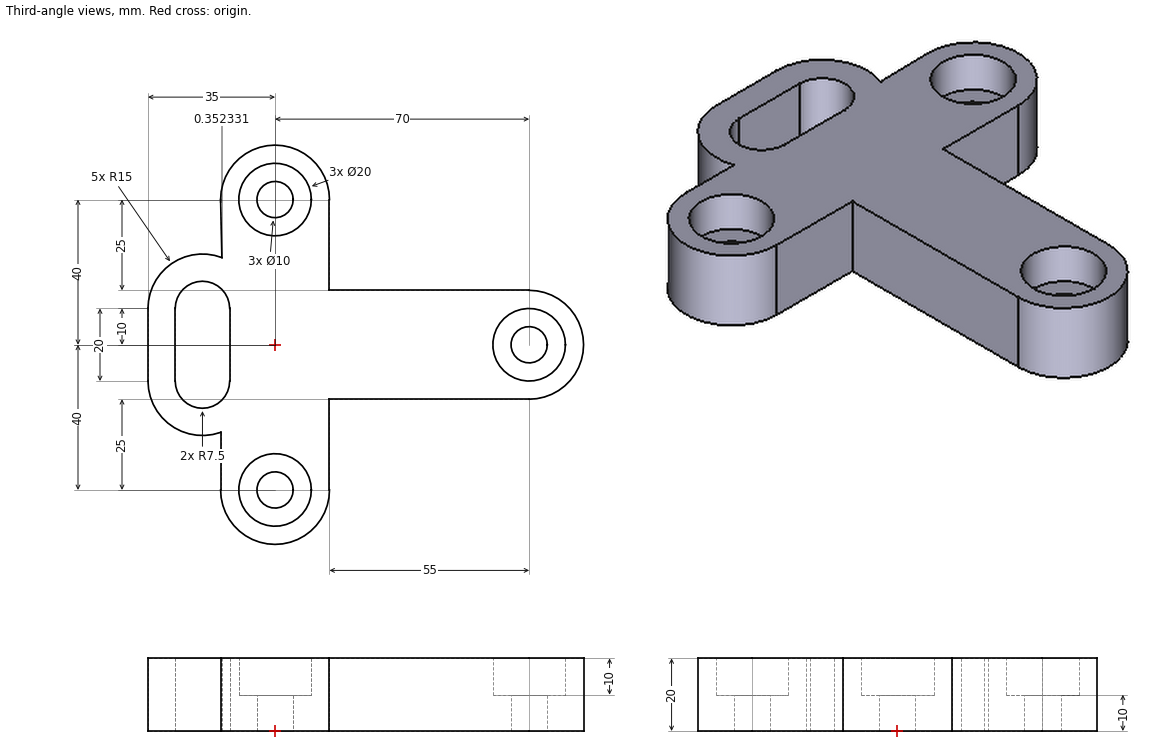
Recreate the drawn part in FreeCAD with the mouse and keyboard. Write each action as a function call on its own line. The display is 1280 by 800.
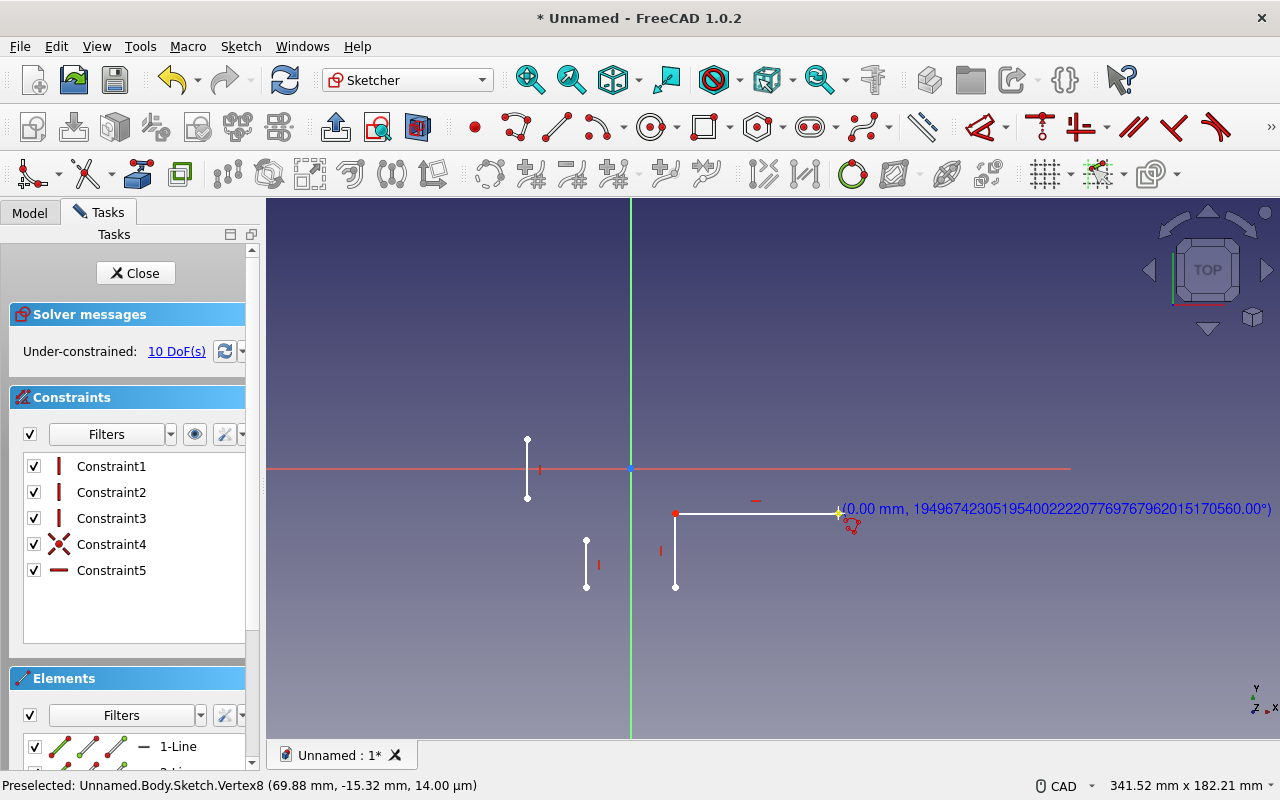
click(838, 424)
click(675, 424)
click(675, 350)
right_click(675, 350)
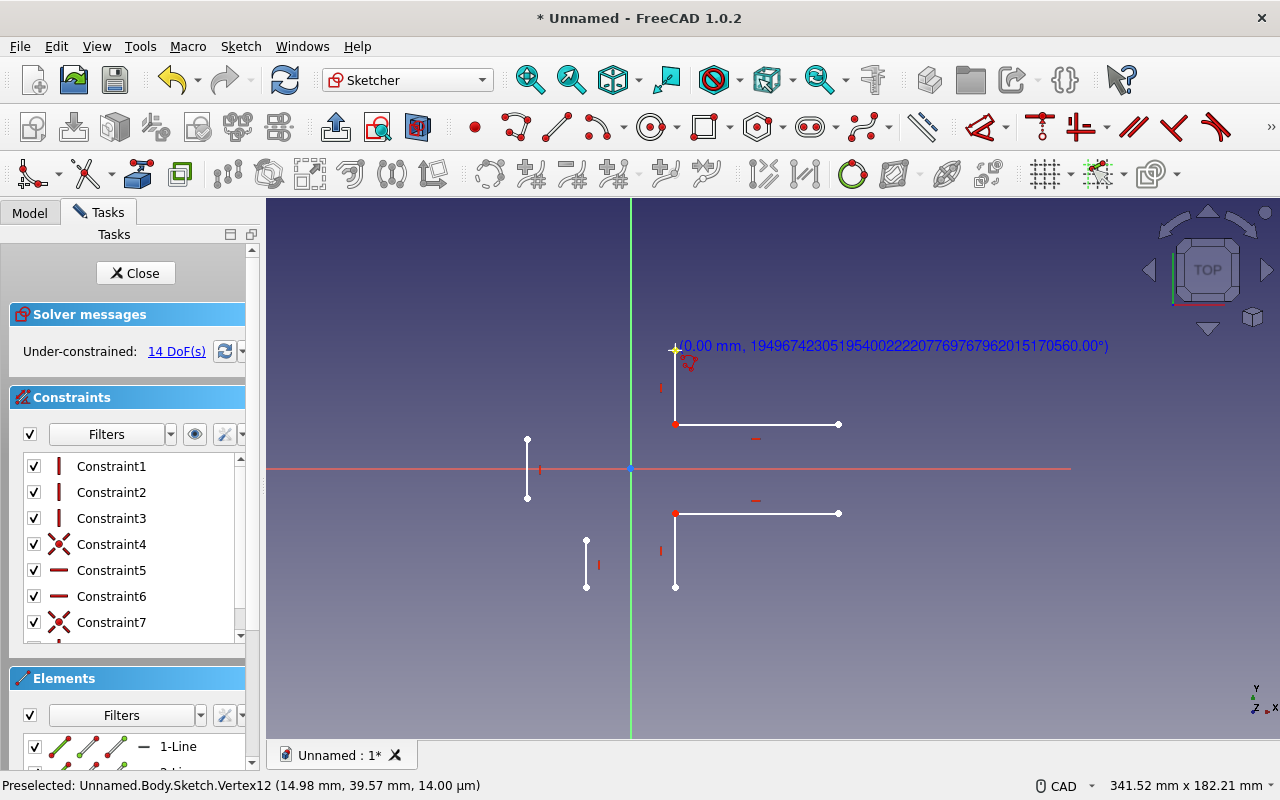
click(557, 128)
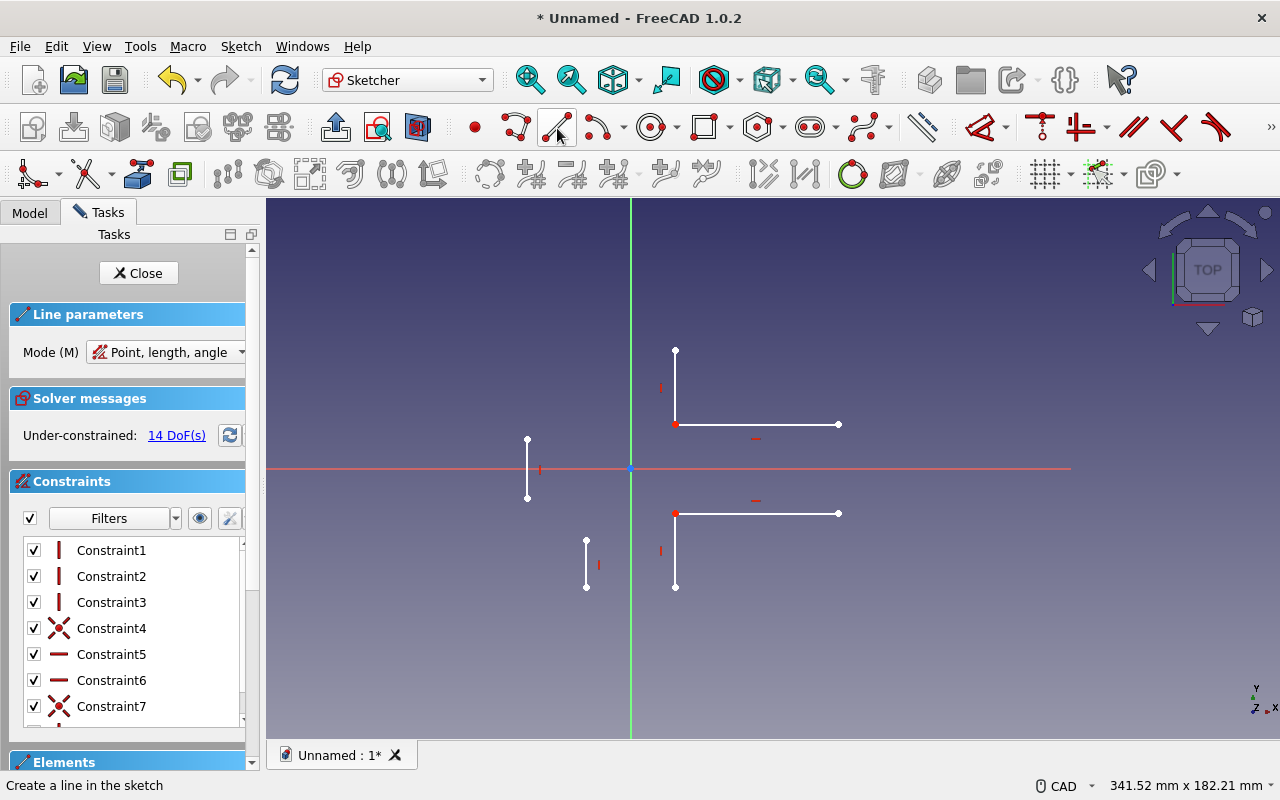
click(586, 350)
click(590, 397)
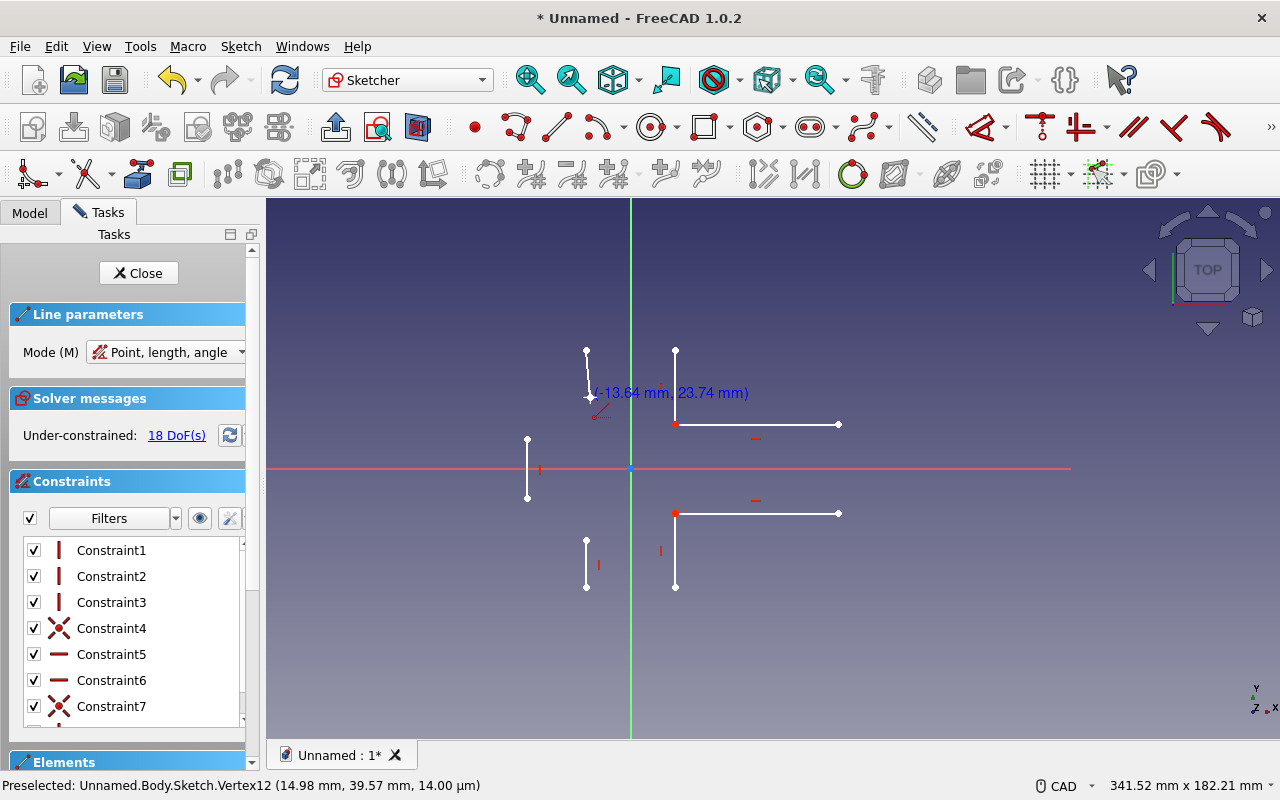
click(624, 128)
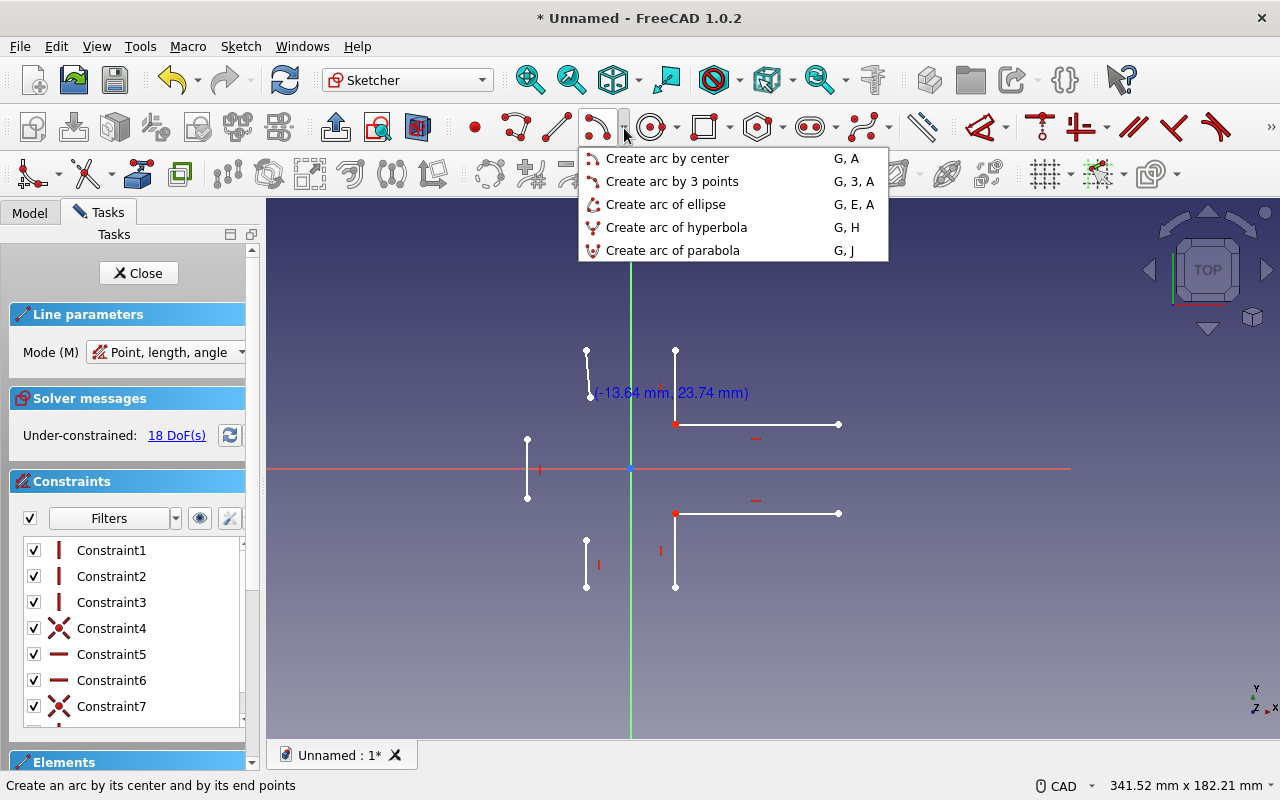
click(734, 182)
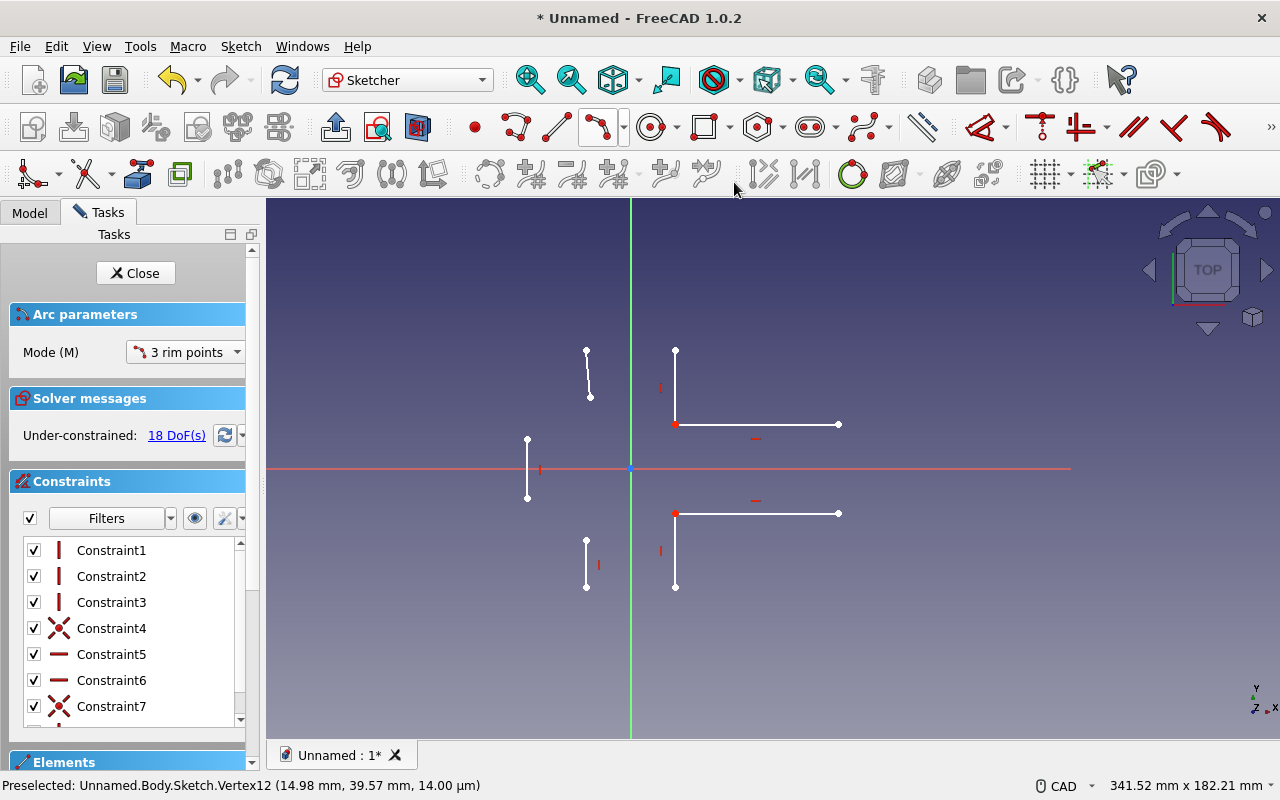
click(527, 499)
click(586, 541)
click(545, 535)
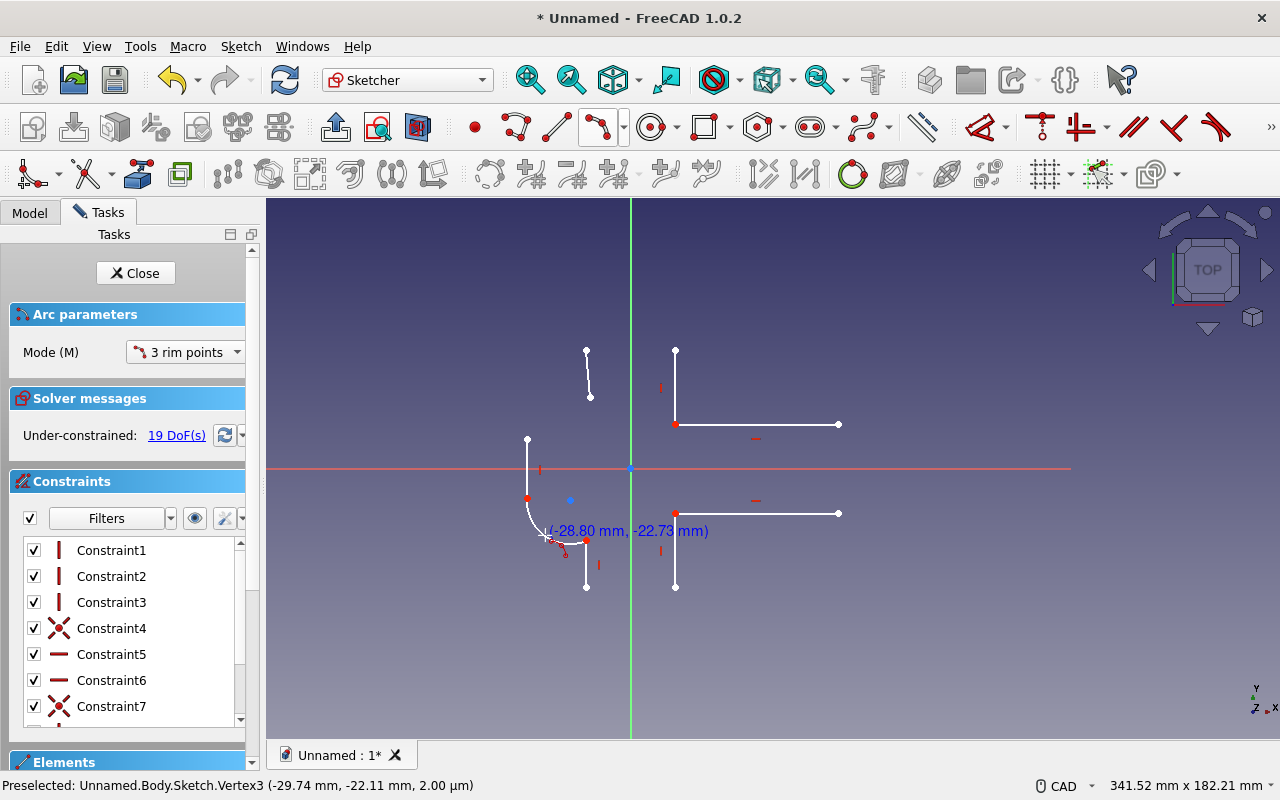
click(586, 588)
click(675, 588)
click(604, 623)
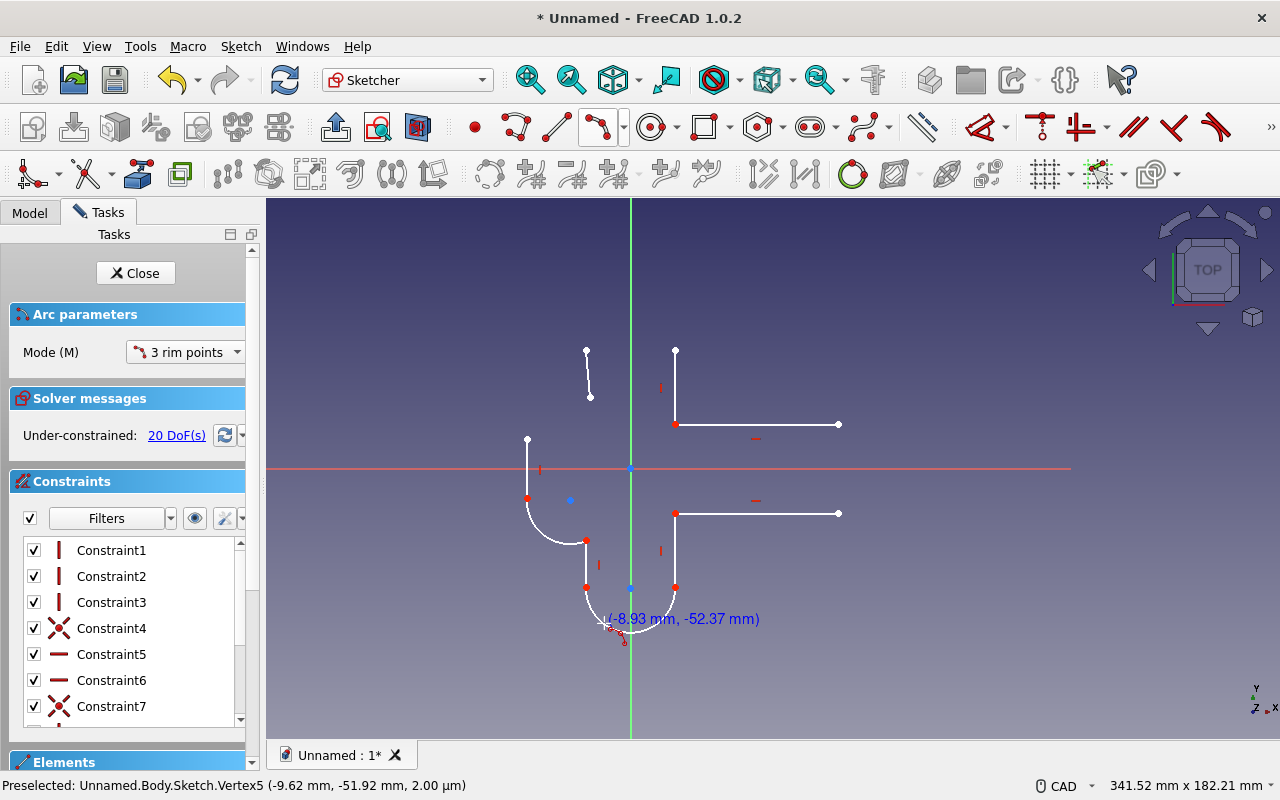
click(838, 514)
click(838, 425)
click(874, 495)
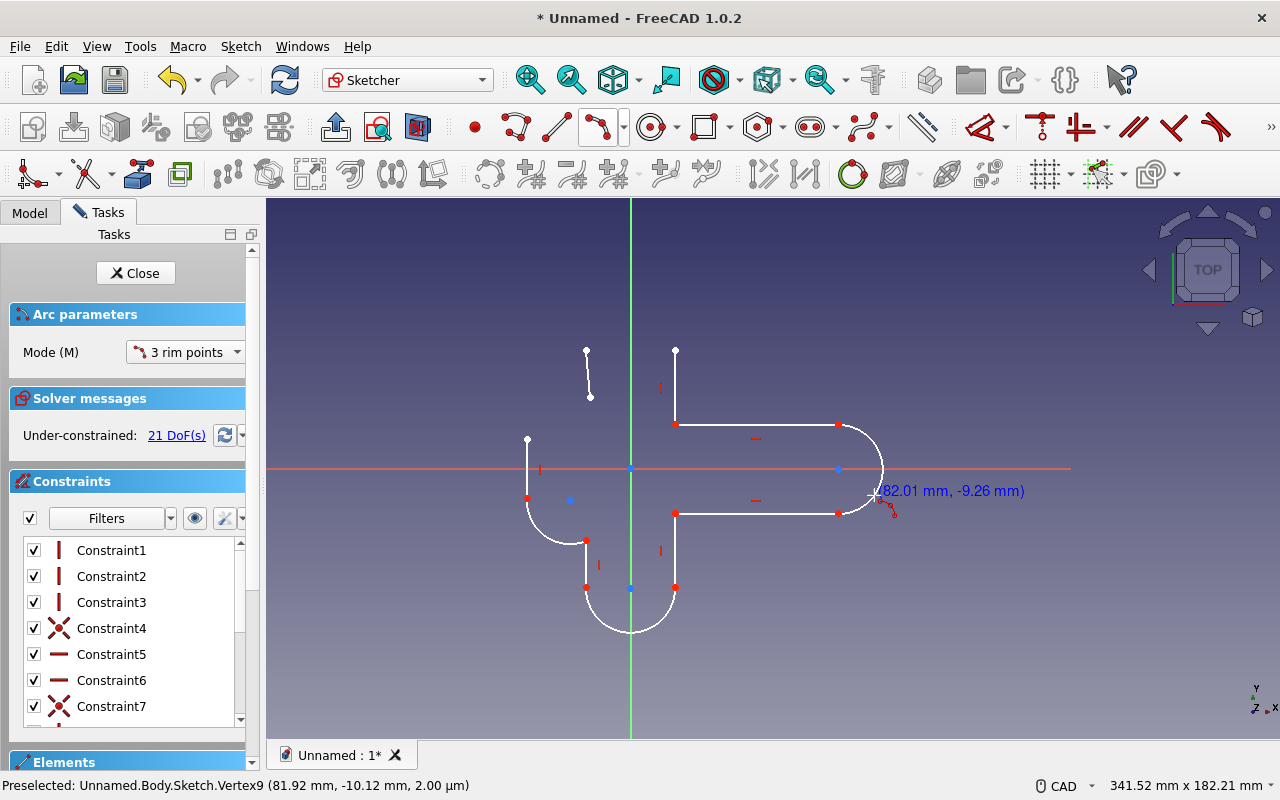
click(675, 351)
click(586, 351)
click(657, 314)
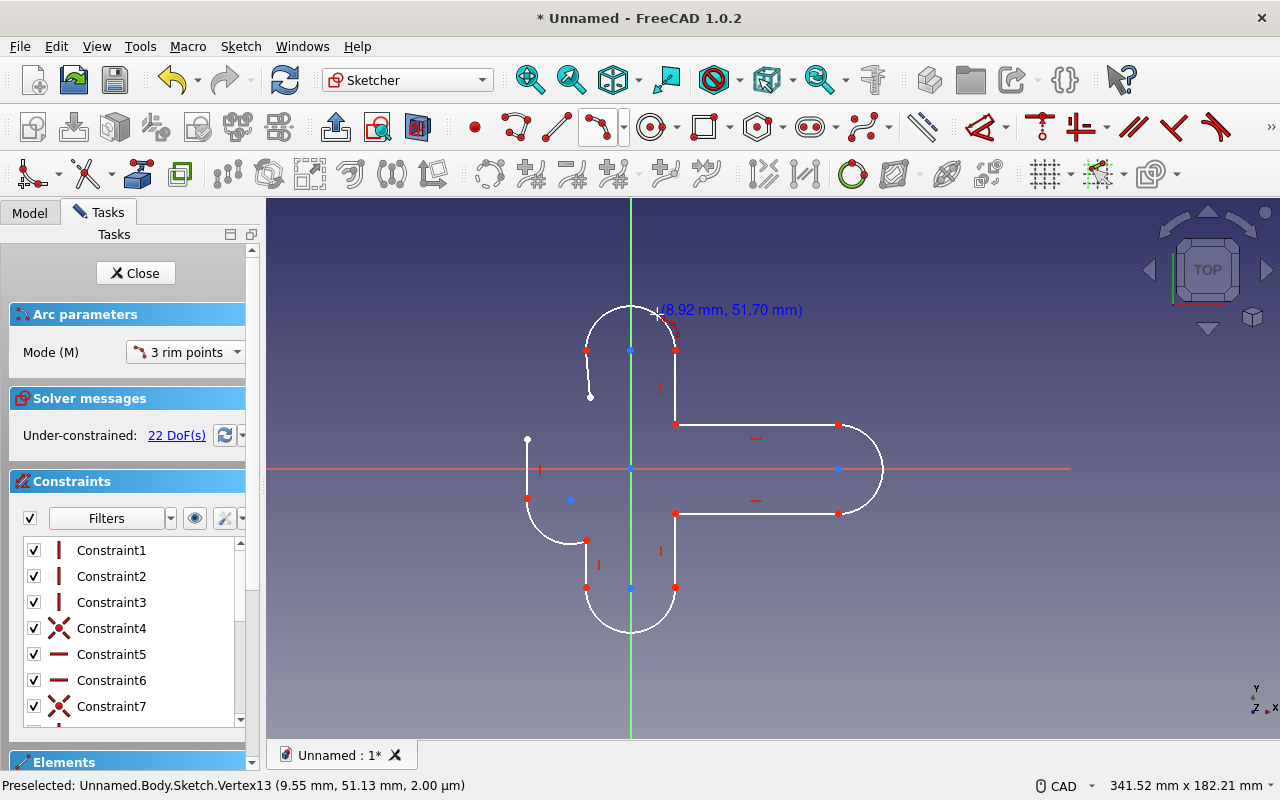
click(590, 398)
click(527, 440)
click(546, 402)